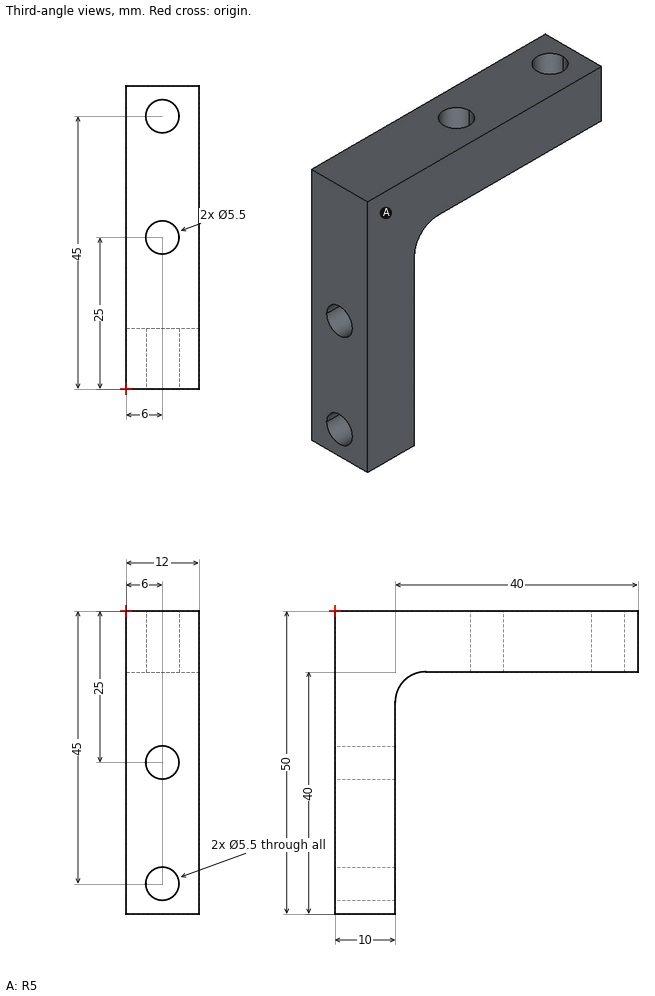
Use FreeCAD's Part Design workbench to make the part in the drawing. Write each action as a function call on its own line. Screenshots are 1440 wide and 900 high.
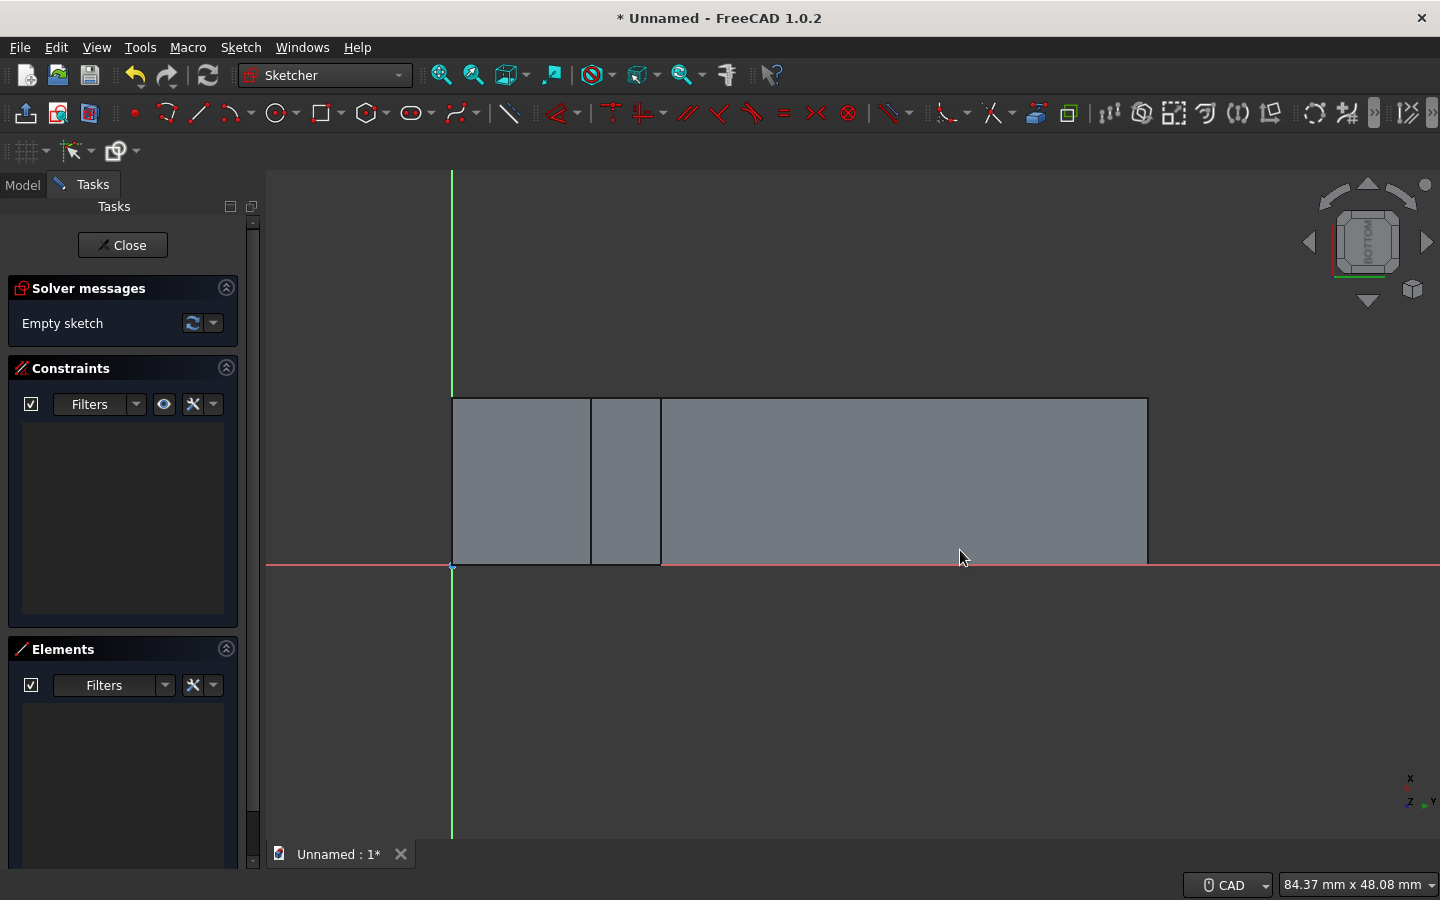
click(276, 114)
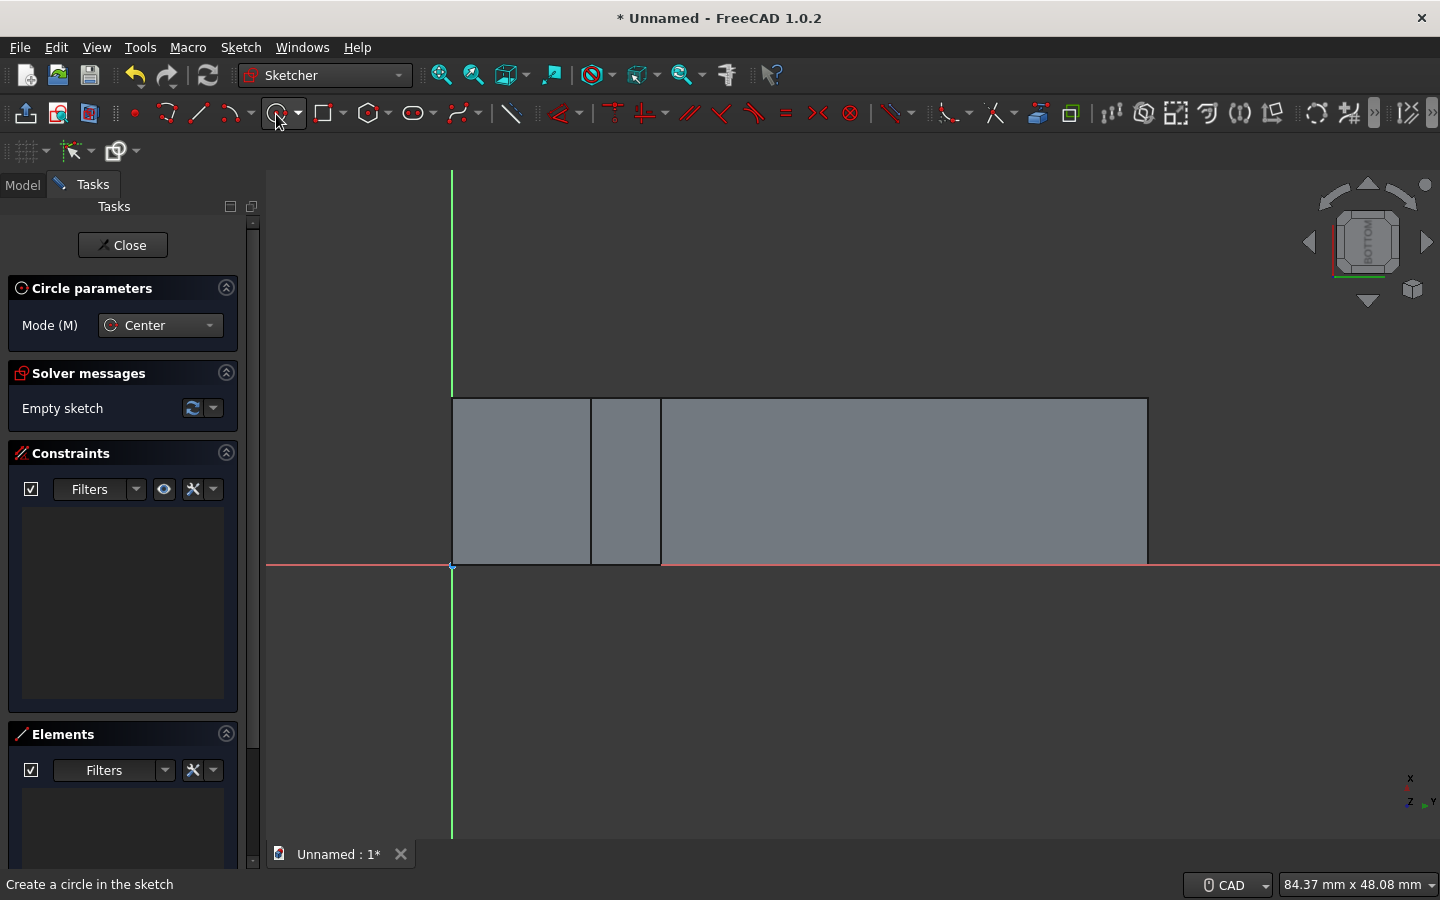
click(800, 482)
click(827, 455)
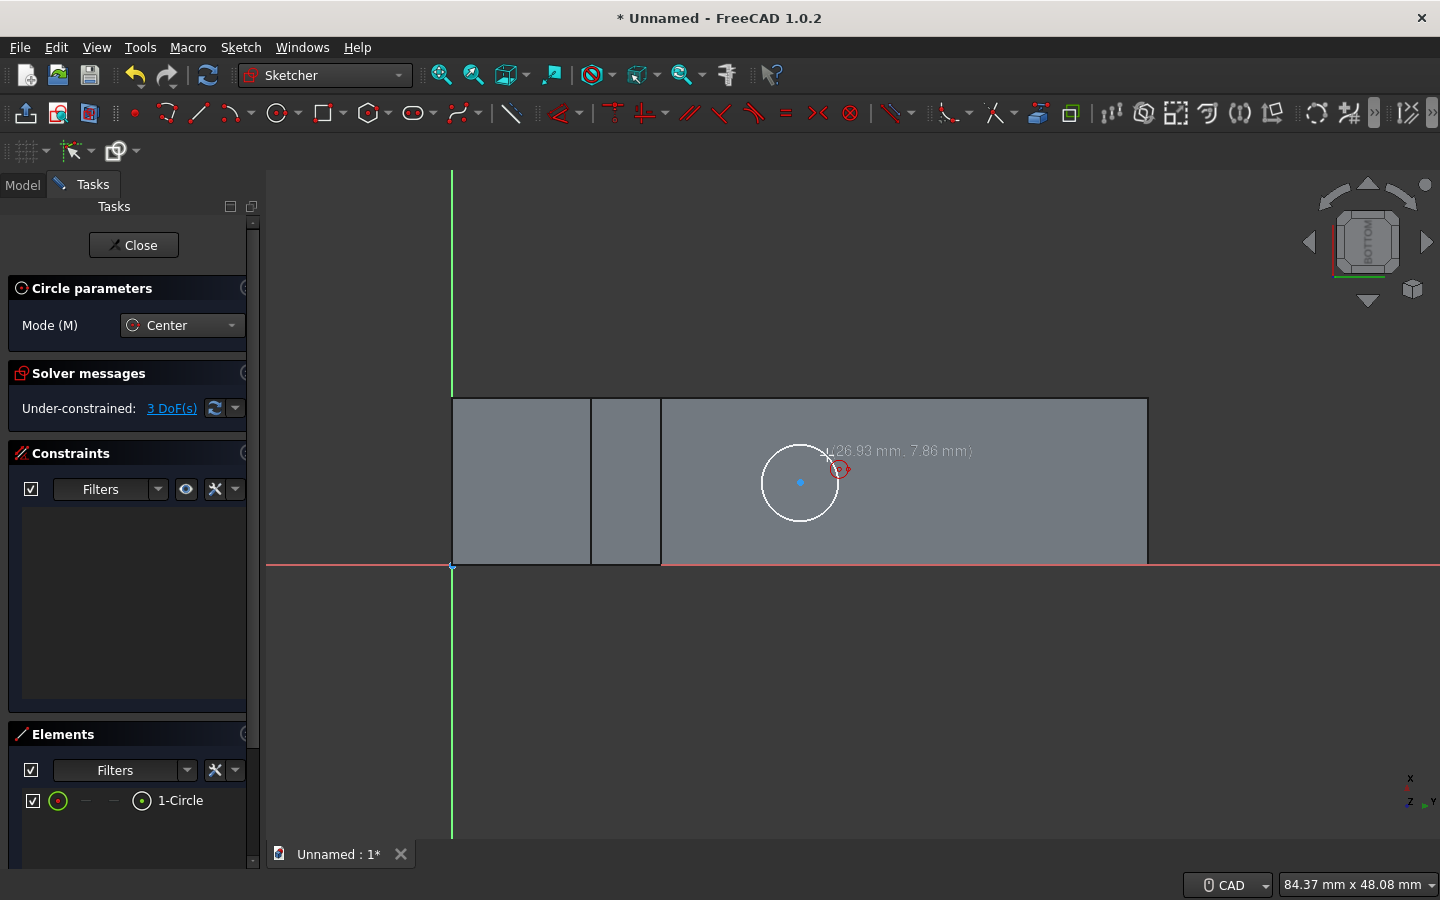
click(1078, 482)
click(1105, 455)
key(Escape)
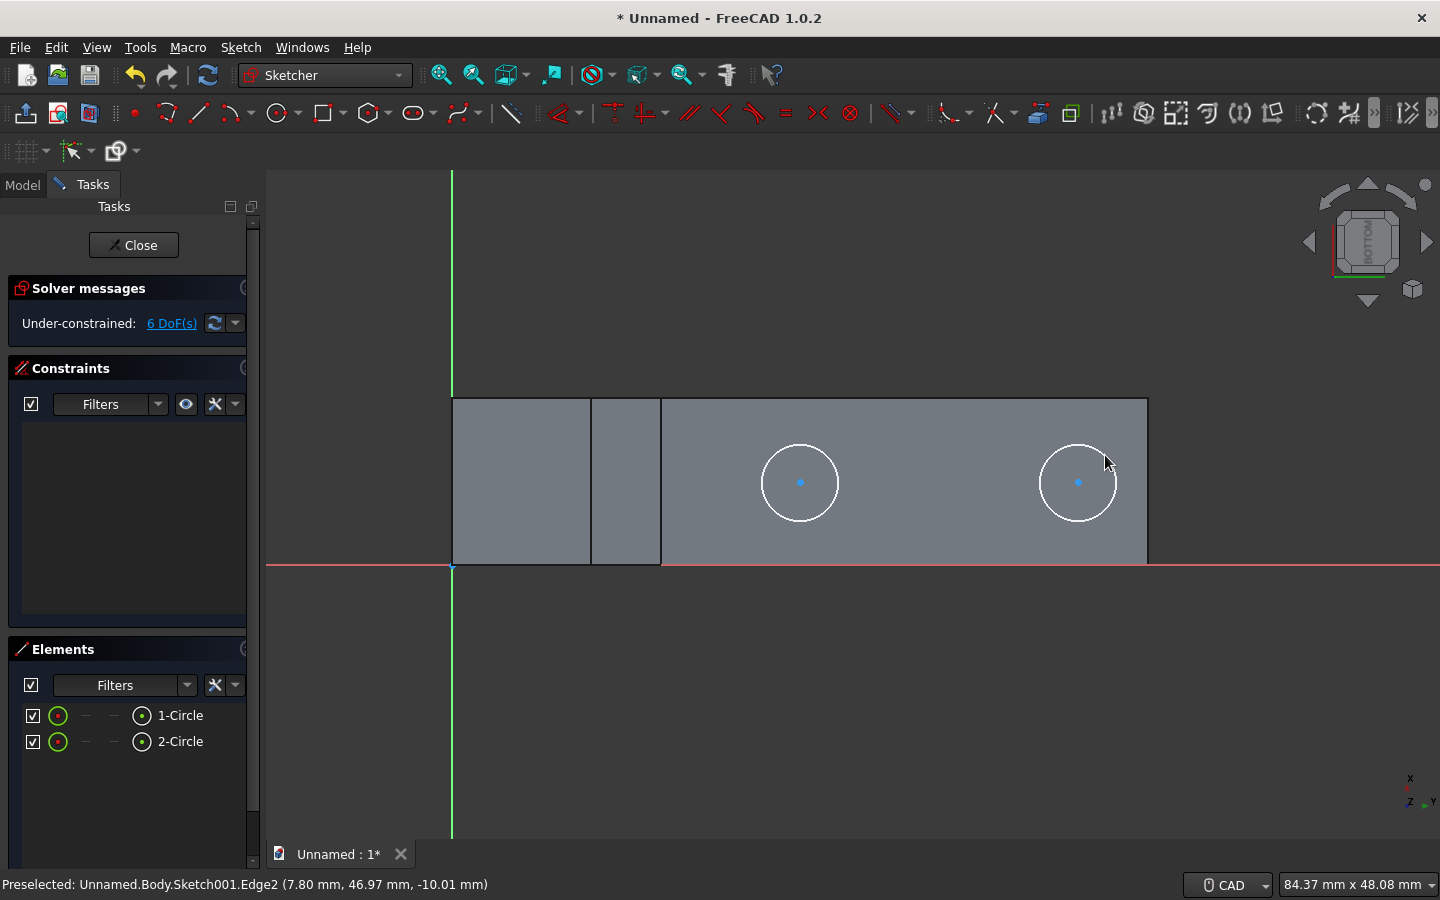
click(827, 456)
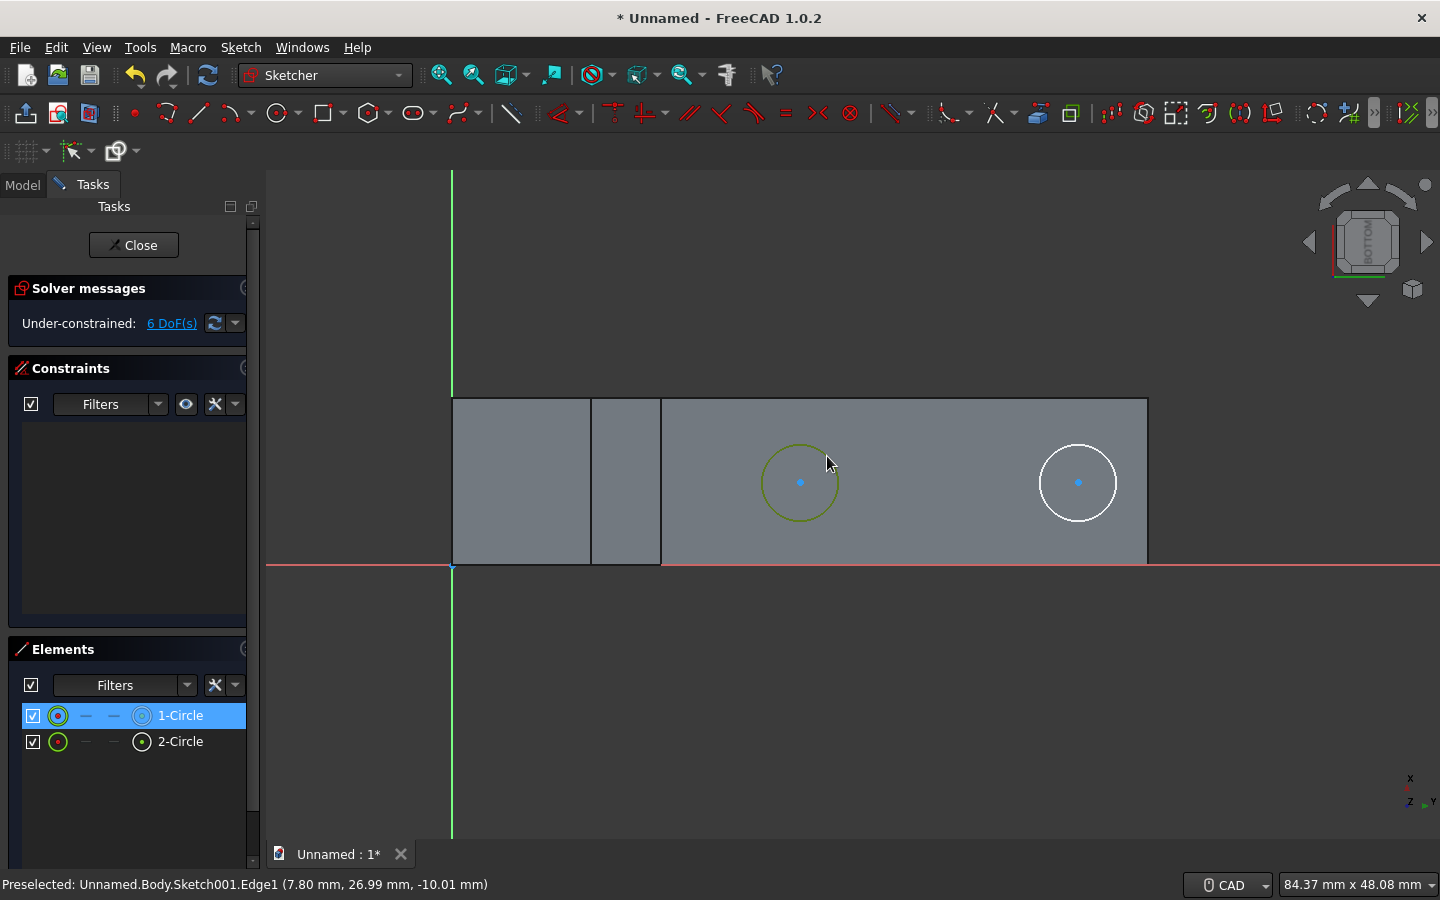
click(1105, 456)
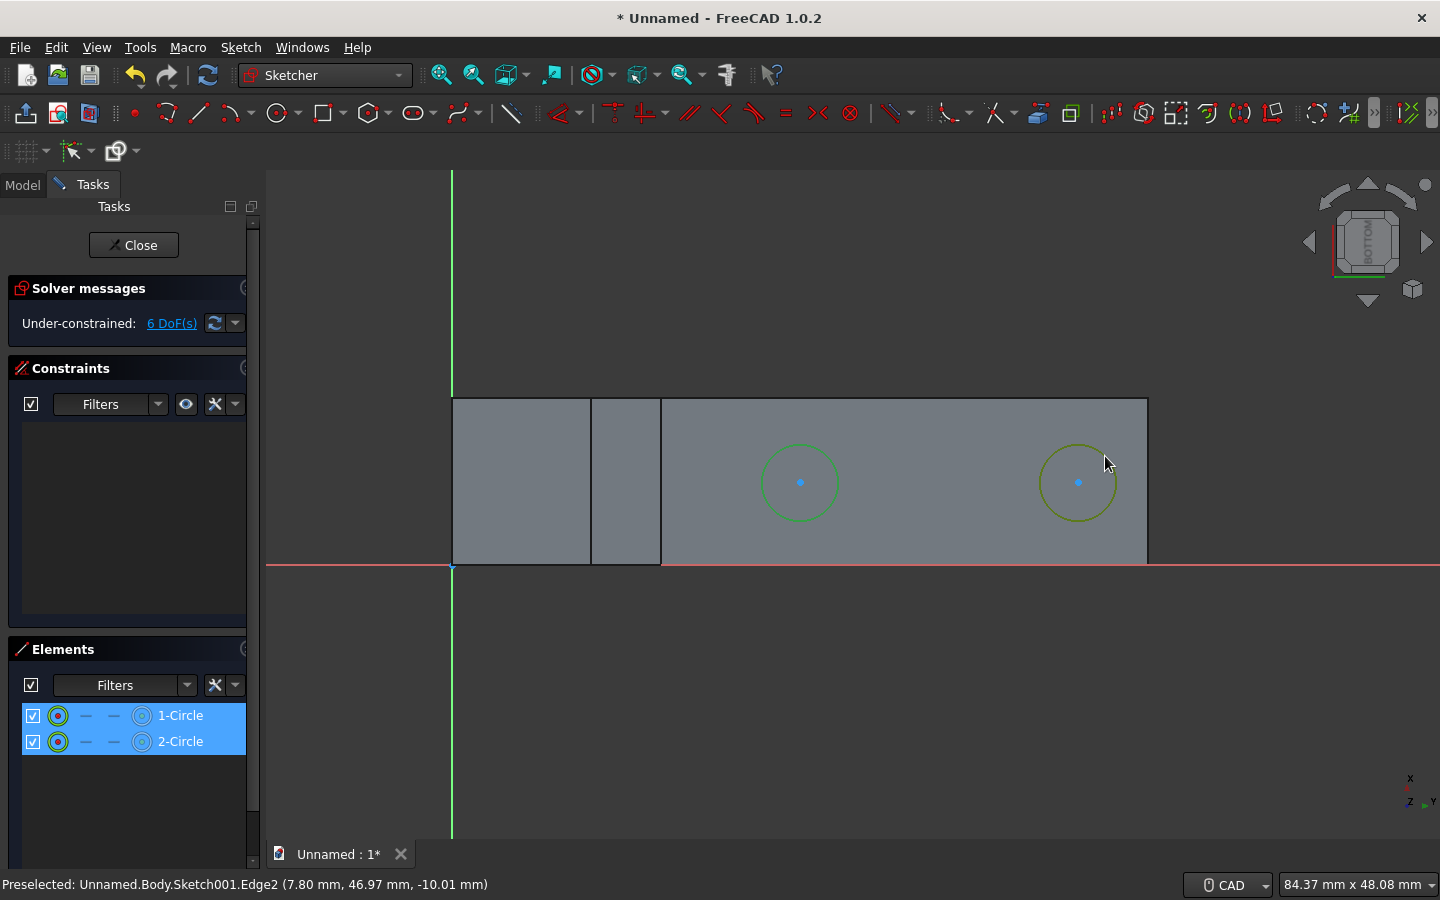
click(786, 114)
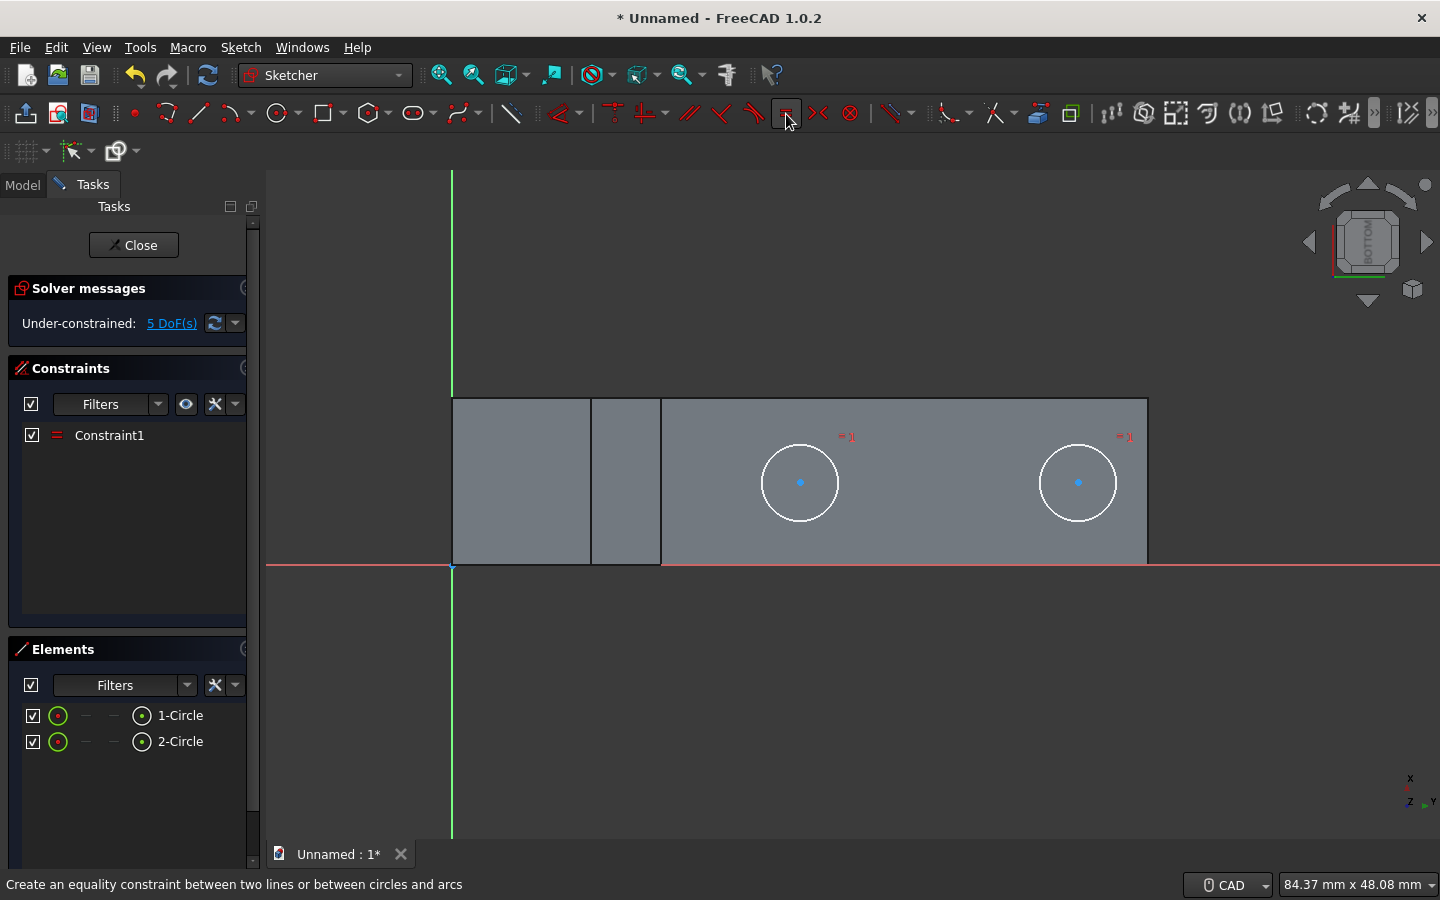
click(558, 114)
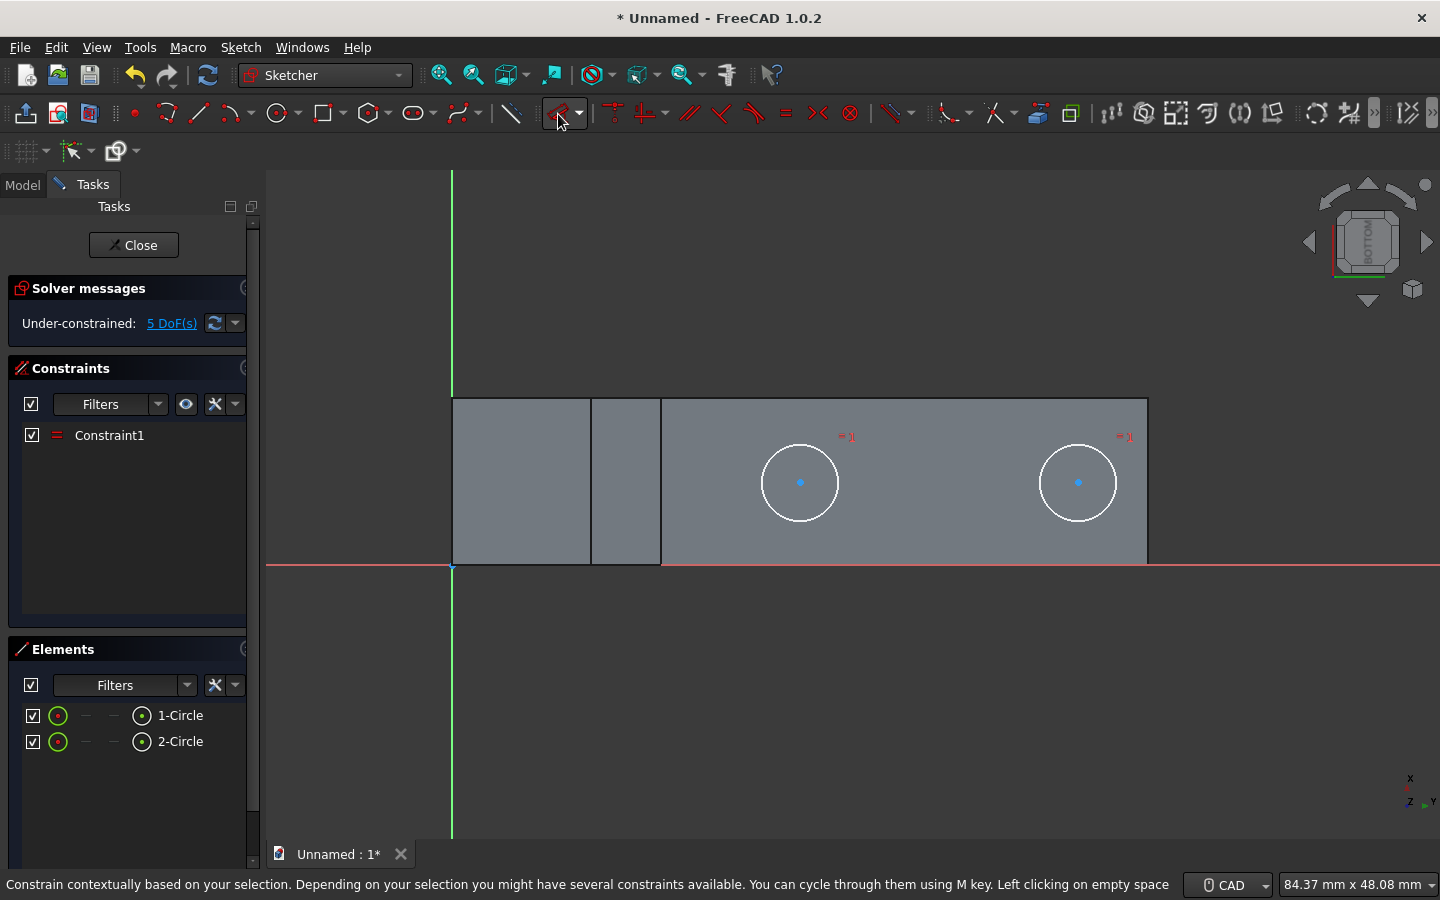
click(827, 456)
click(850, 433)